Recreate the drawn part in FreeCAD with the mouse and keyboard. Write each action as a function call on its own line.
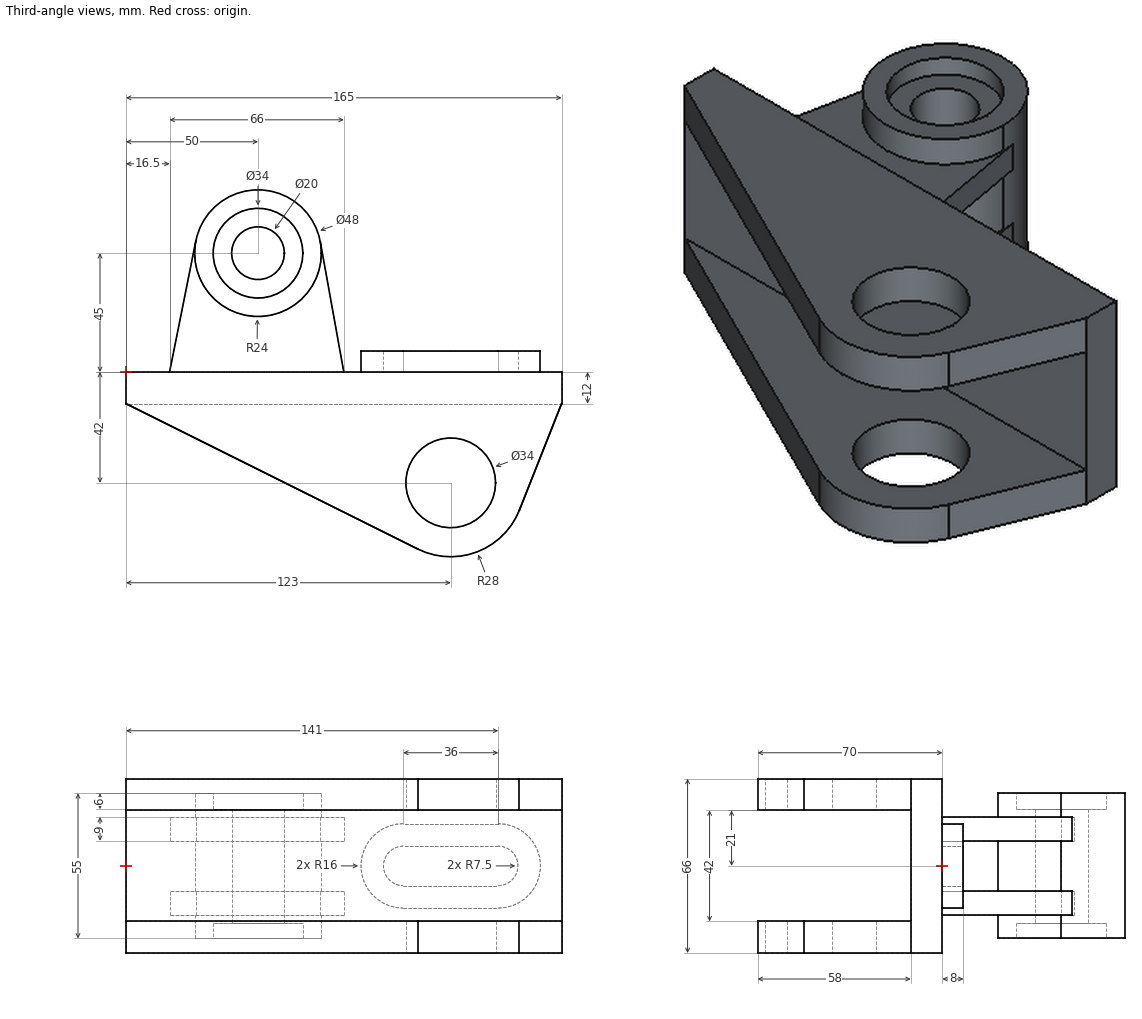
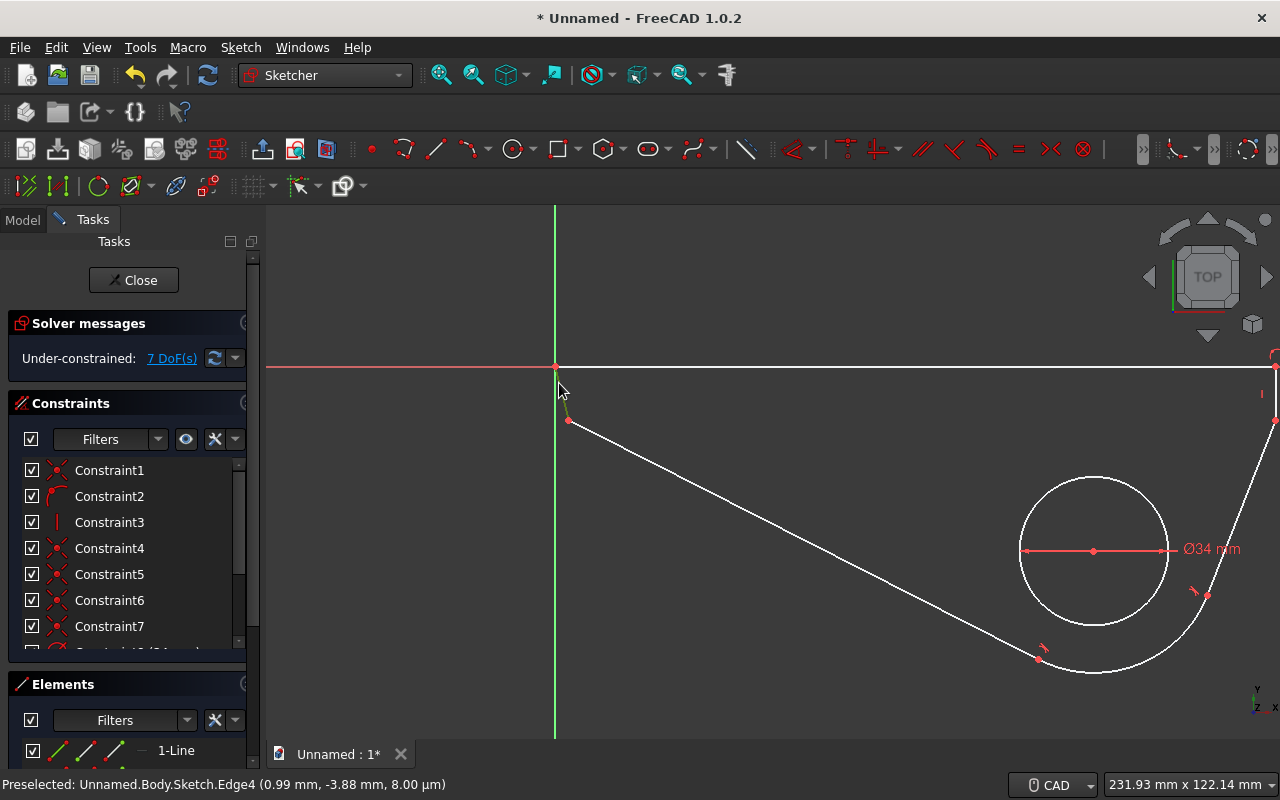
key(v)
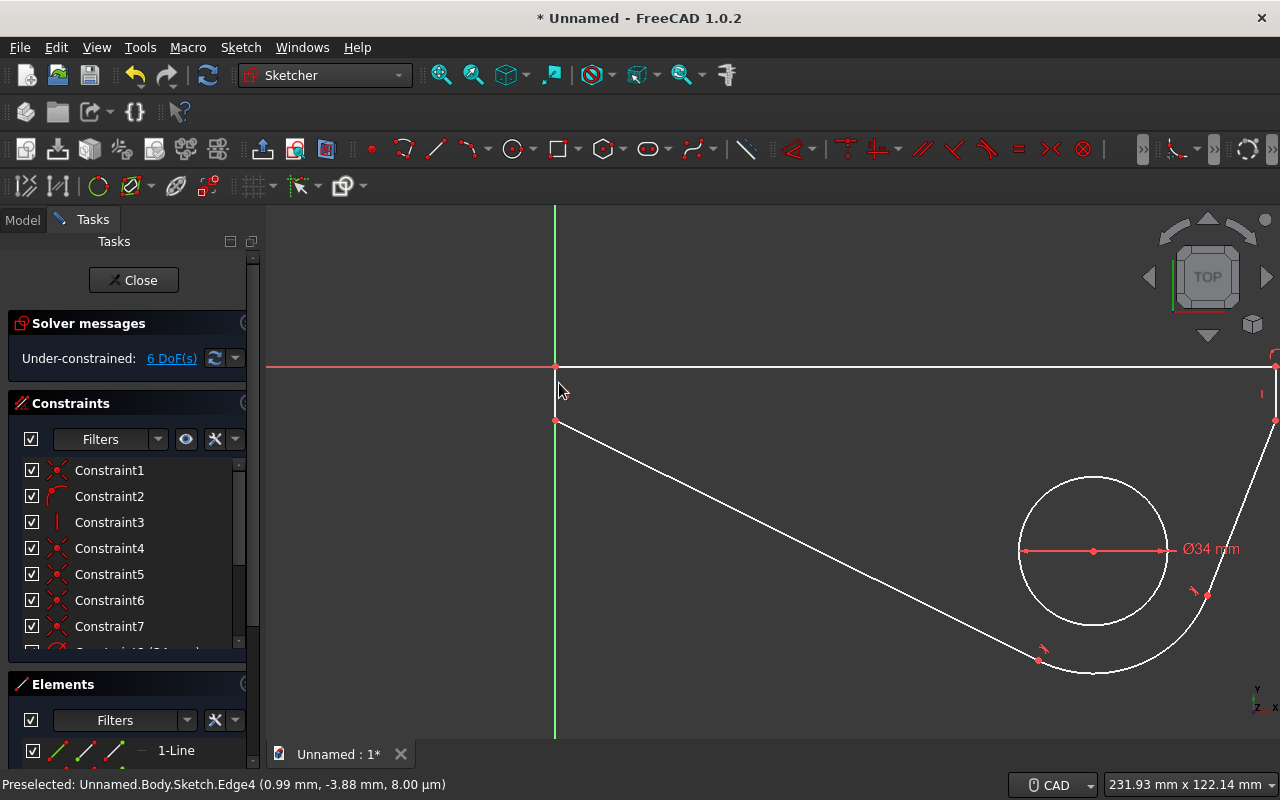
click(792, 150)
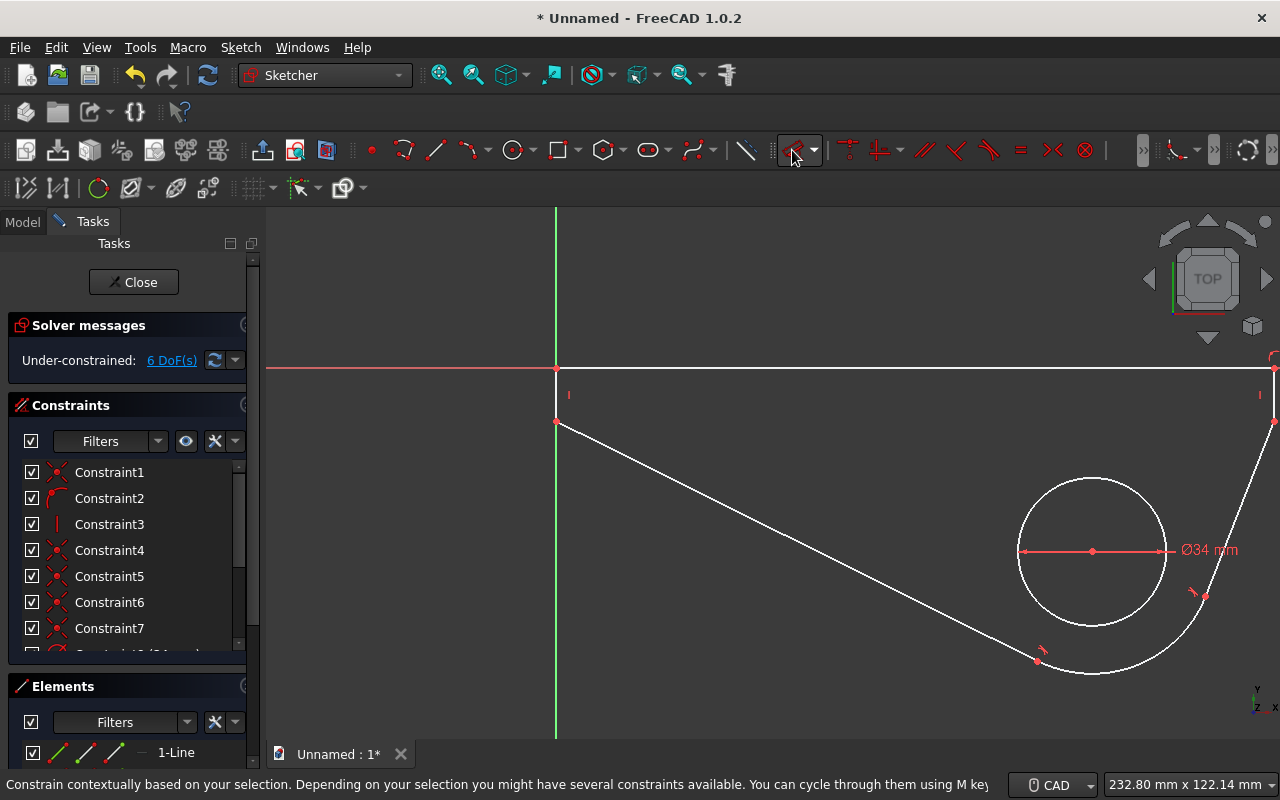
click(1096, 674)
click(1097, 706)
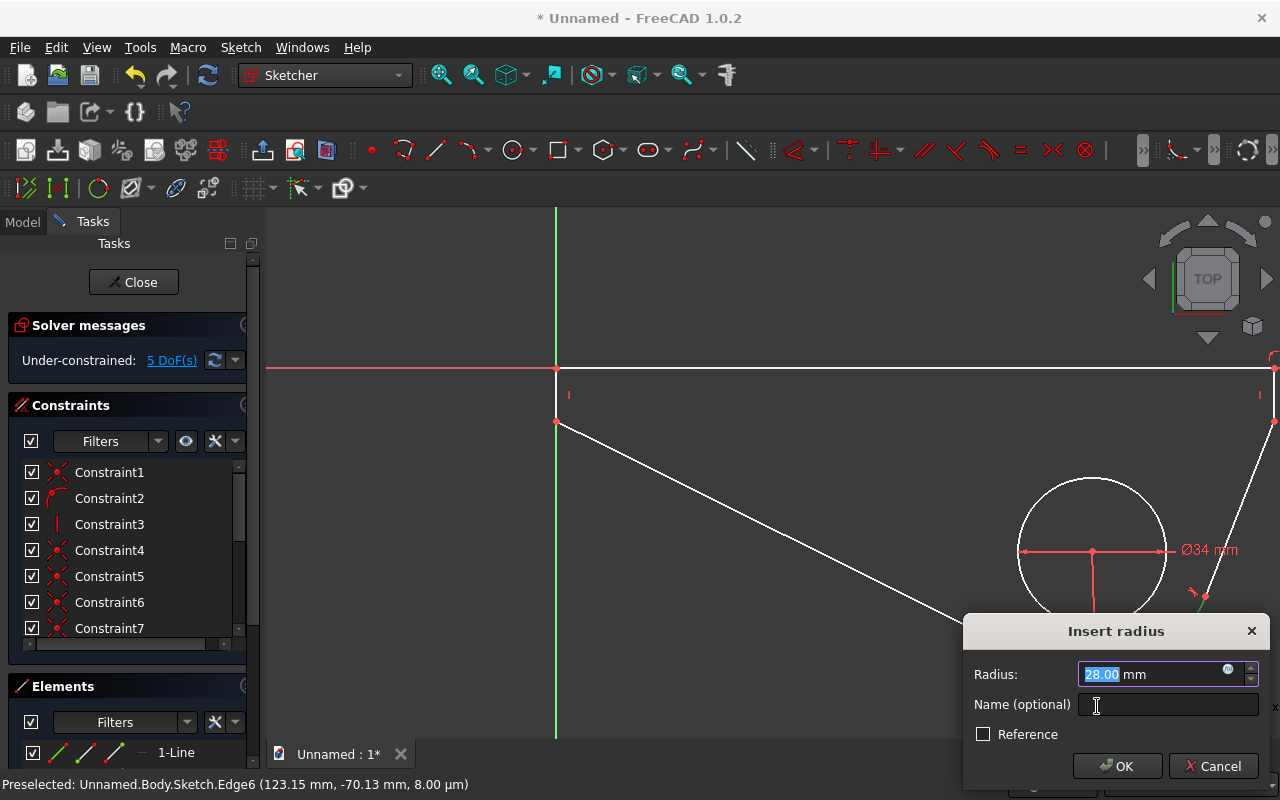
text(28)
key(Return)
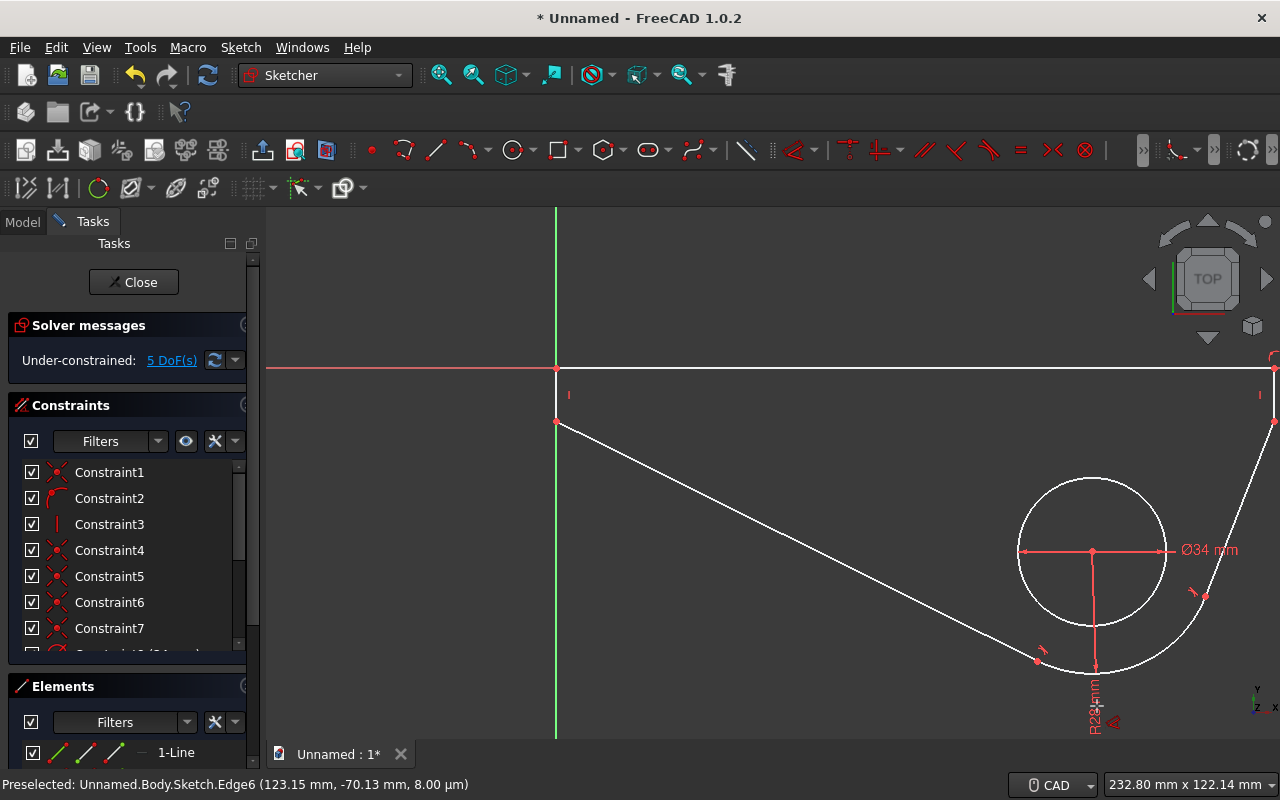
scroll(294, 384, down, 2)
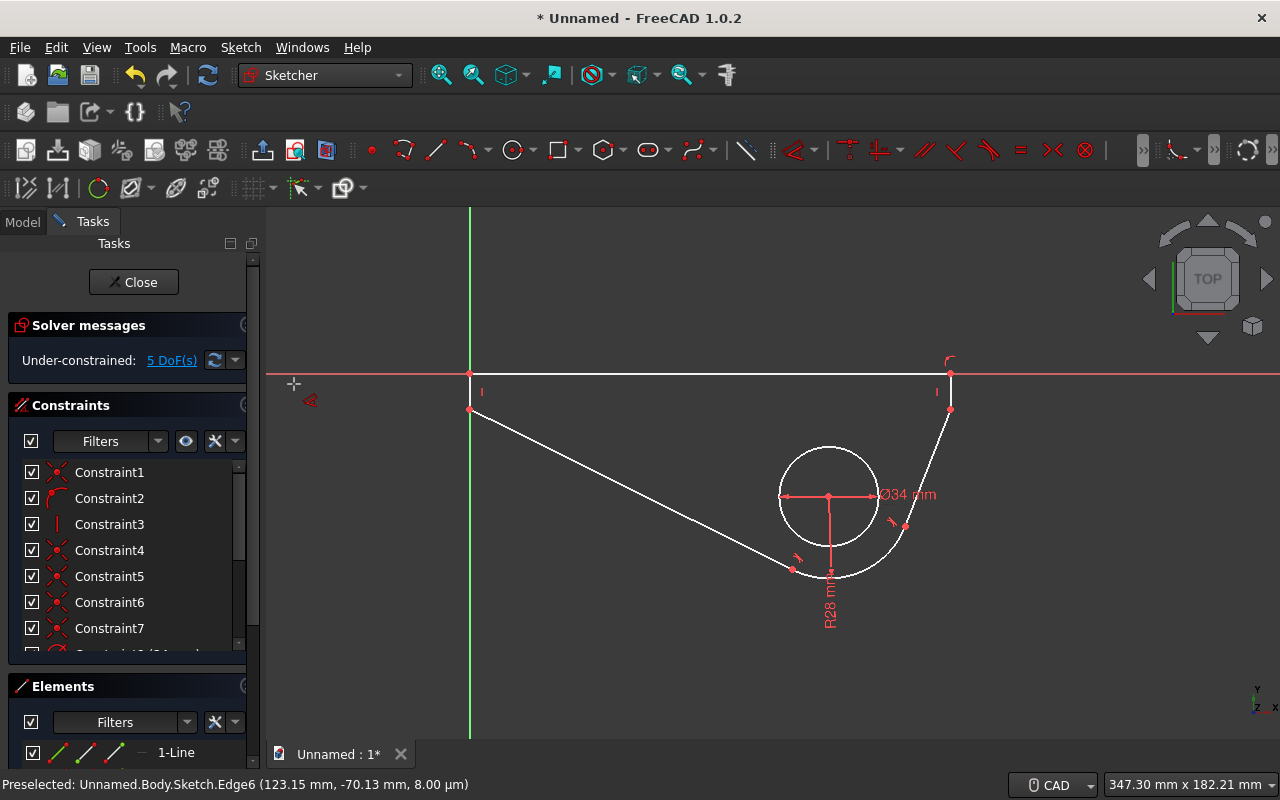
scroll(951, 398, up, 2)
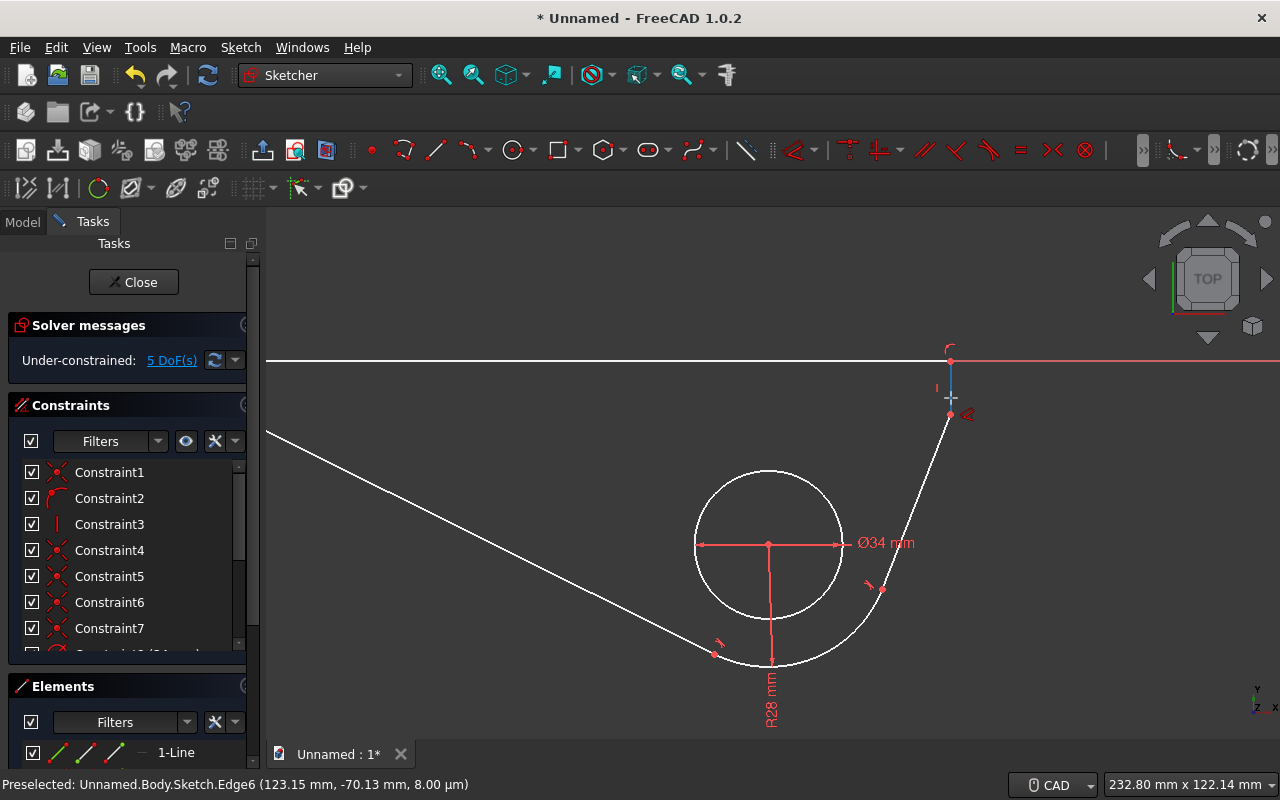
click(951, 399)
click(985, 388)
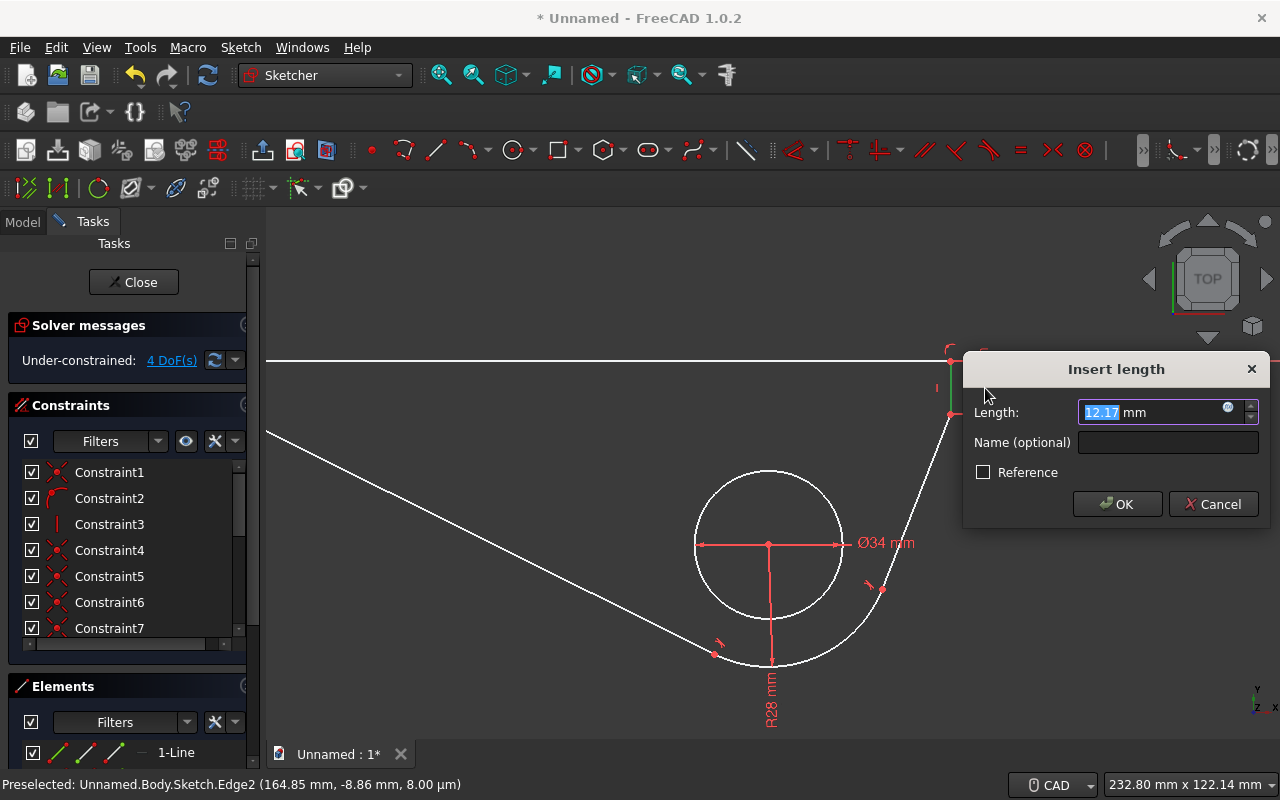
text(12)
key(Return)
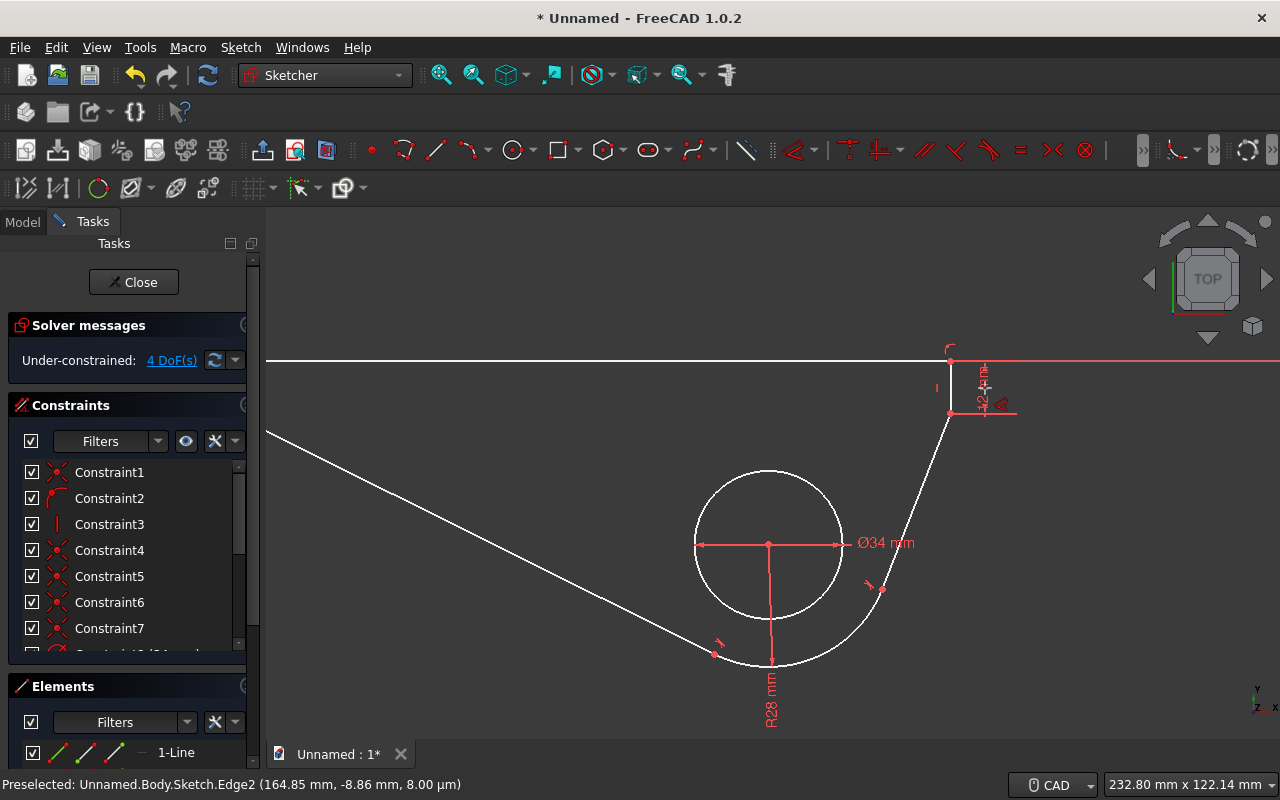
scroll(1115, 307, down, 1)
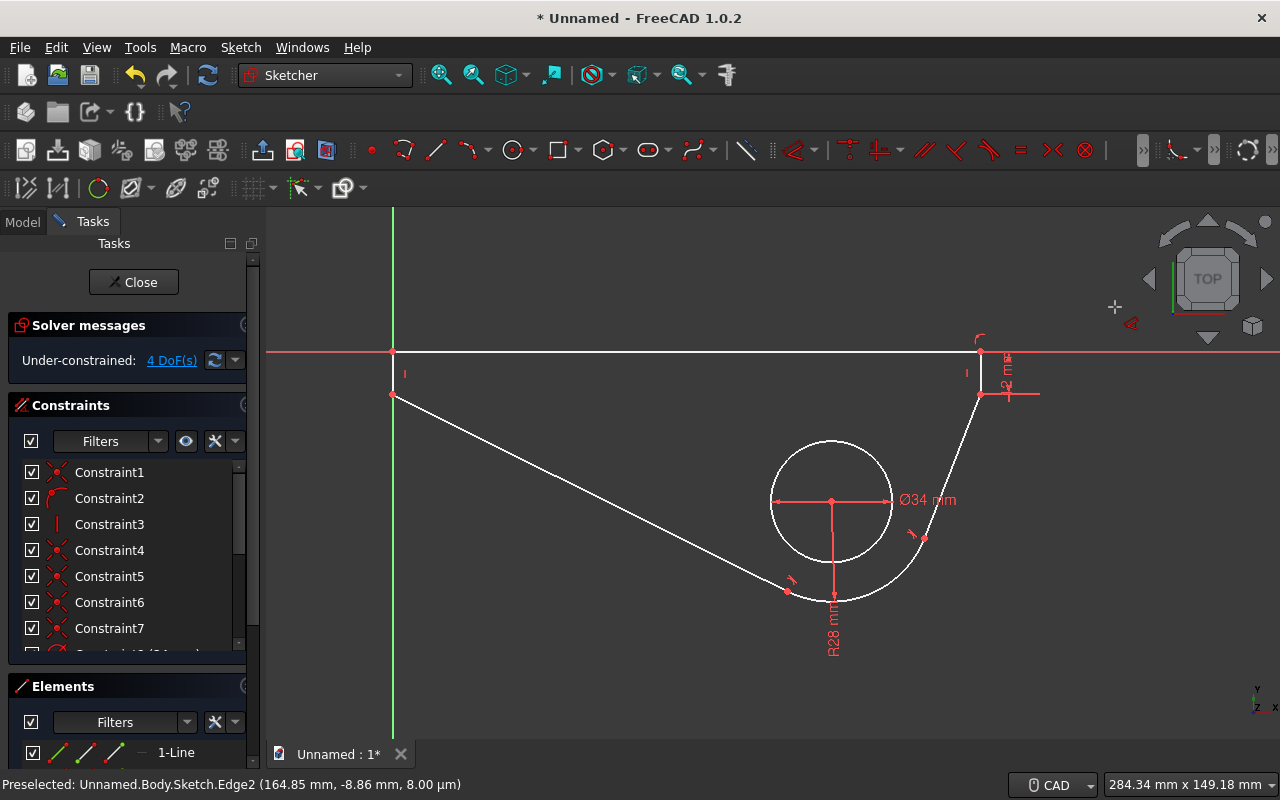
click(393, 365)
click(359, 373)